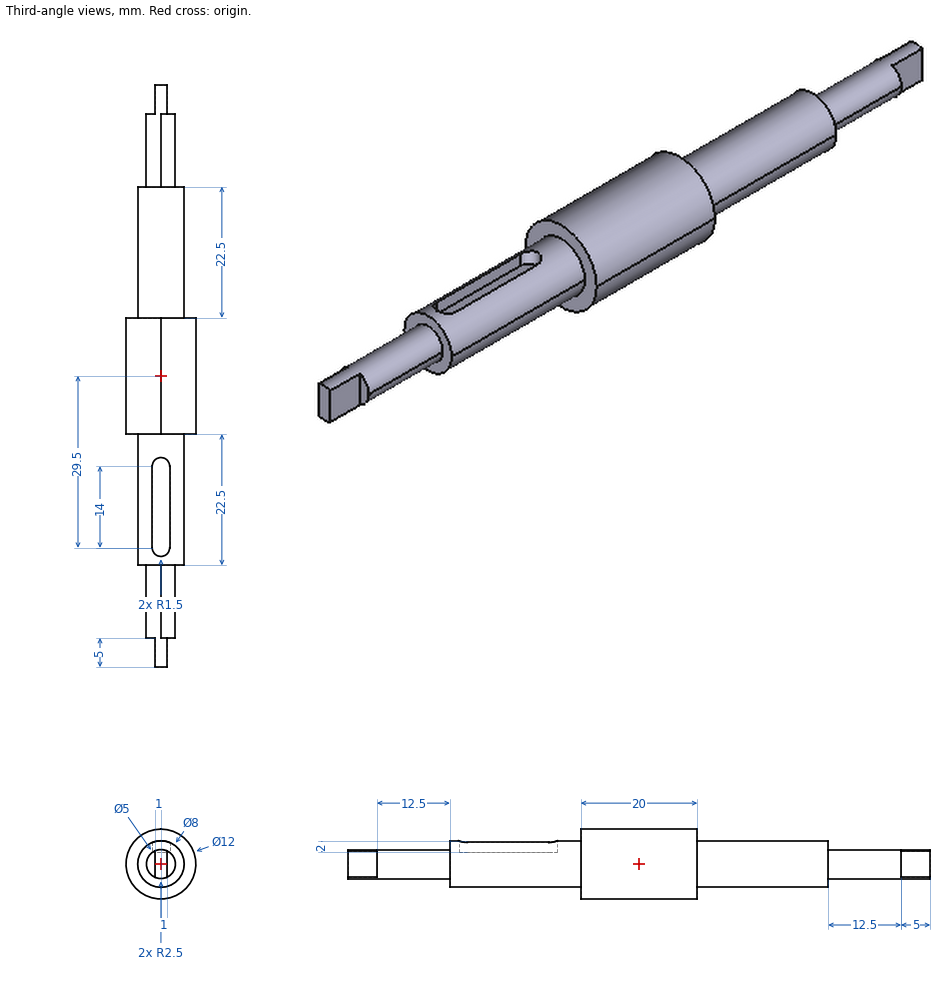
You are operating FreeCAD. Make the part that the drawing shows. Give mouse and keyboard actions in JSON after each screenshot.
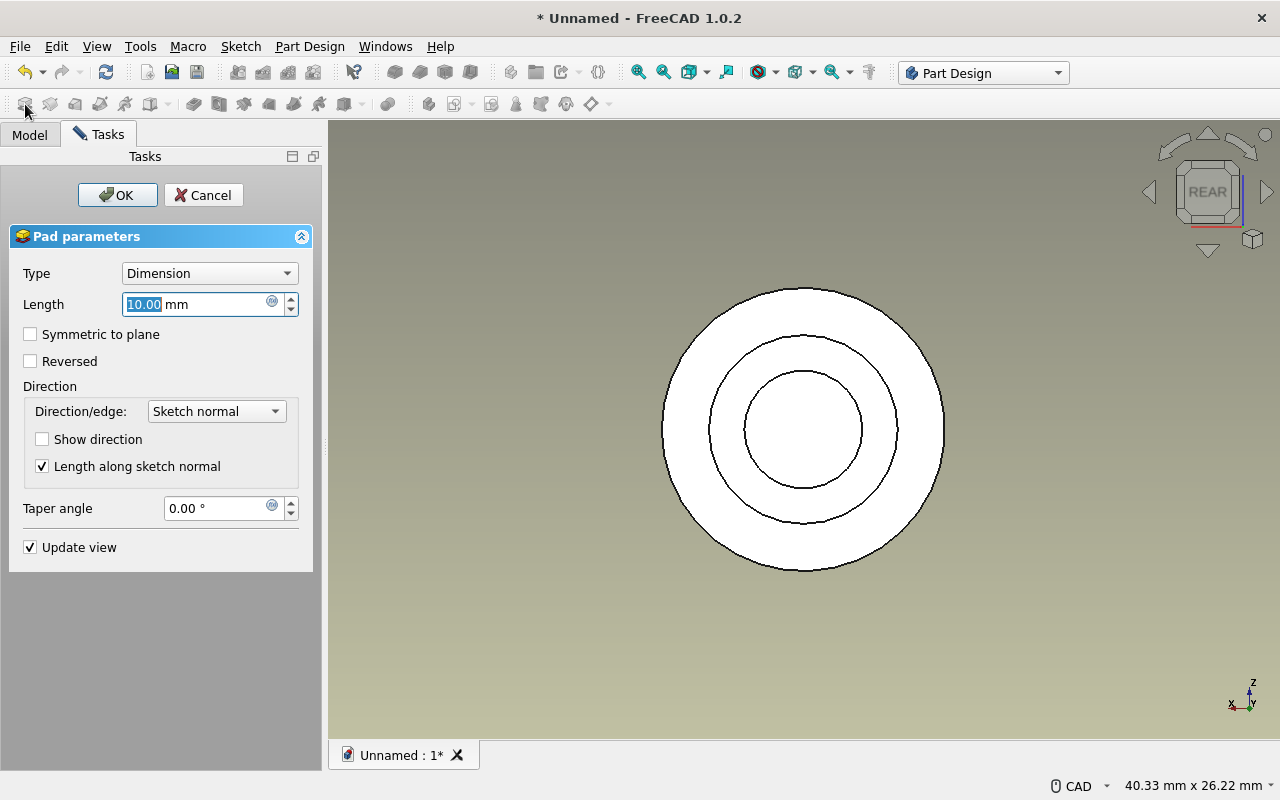
{"action": "type", "text": "22.5"}
{"action": "key", "text": "Tab"}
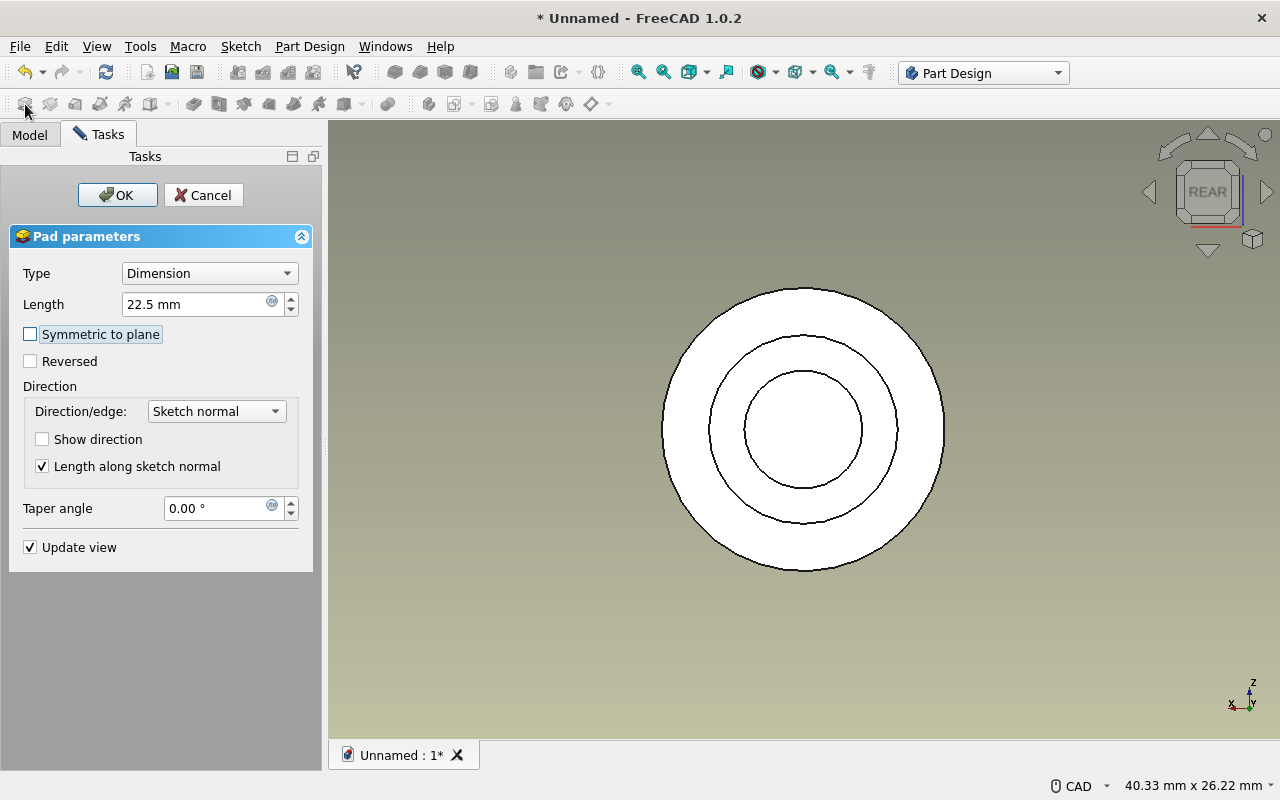
{"action": "left_click", "coordinate": [31, 361]}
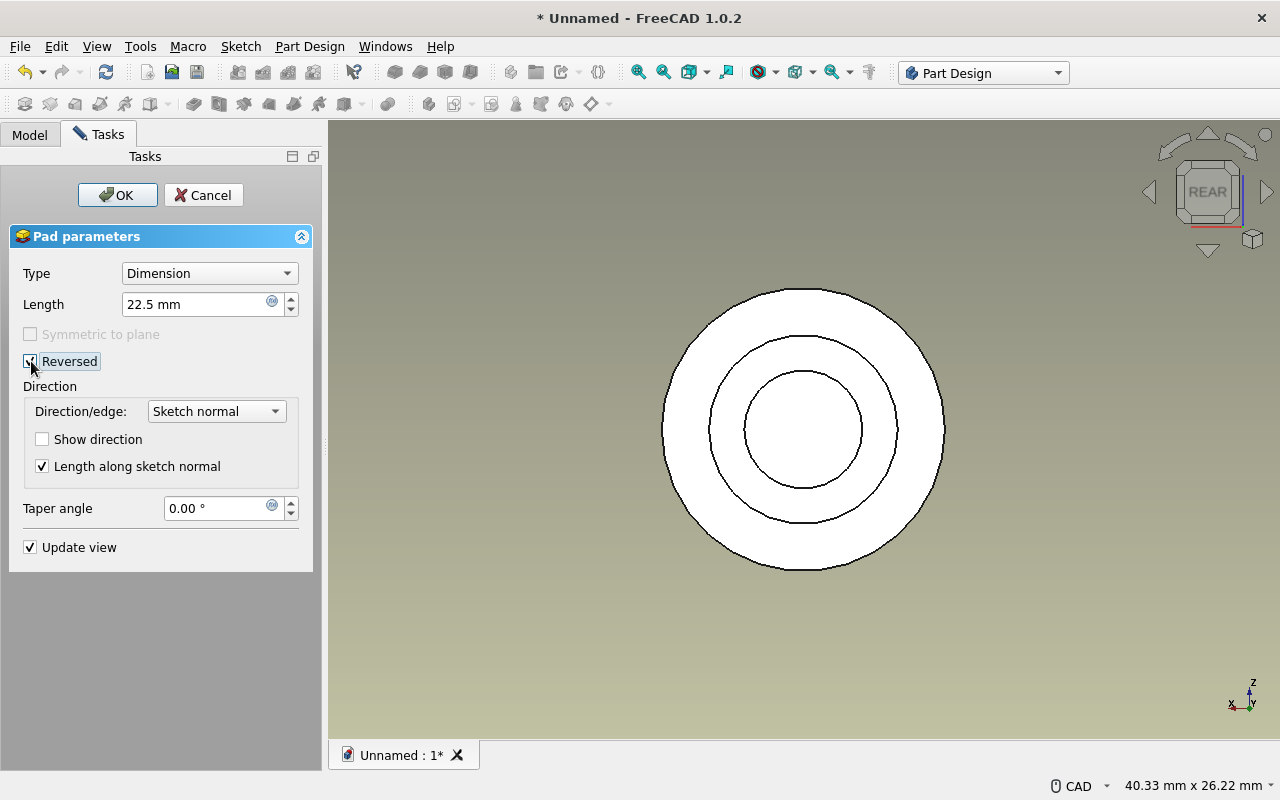
{"action": "left_click", "coordinate": [118, 195]}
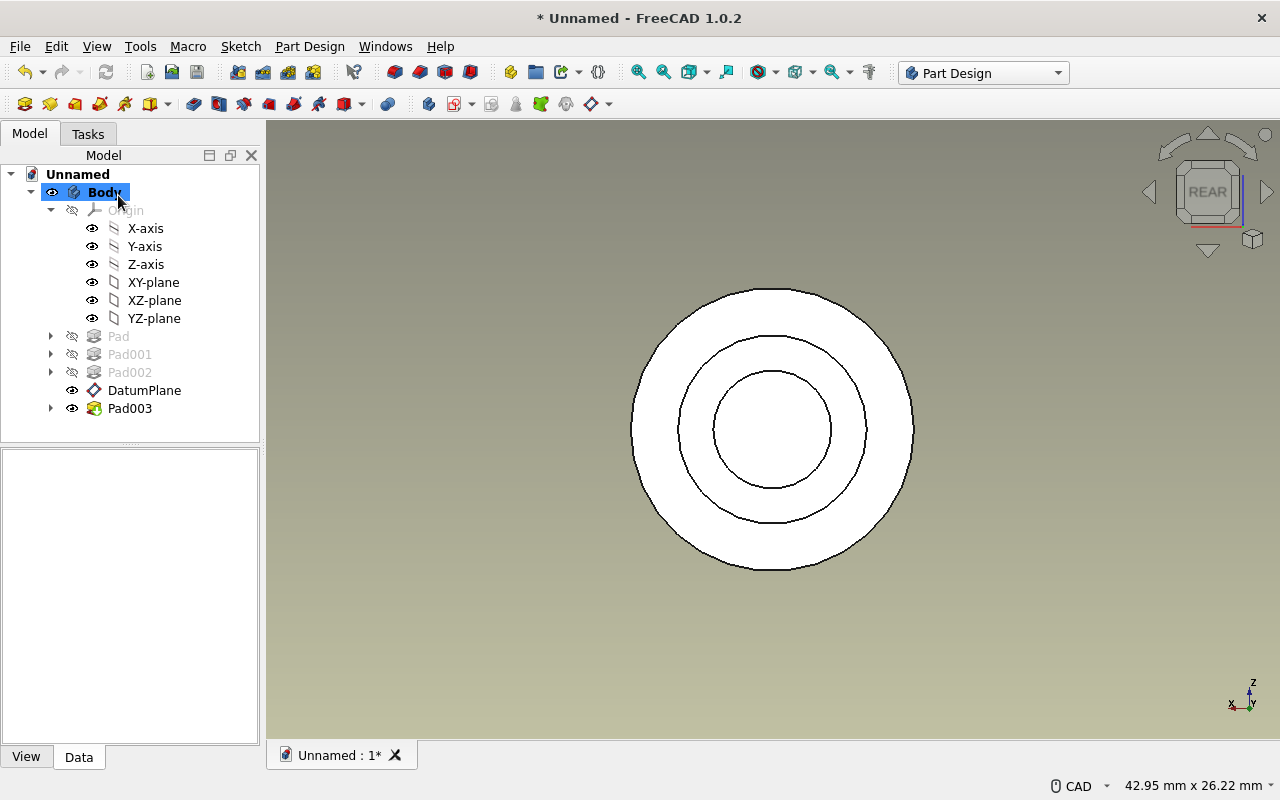
{"action": "left_click", "coordinate": [117, 390]}
{"action": "key", "text": "space"}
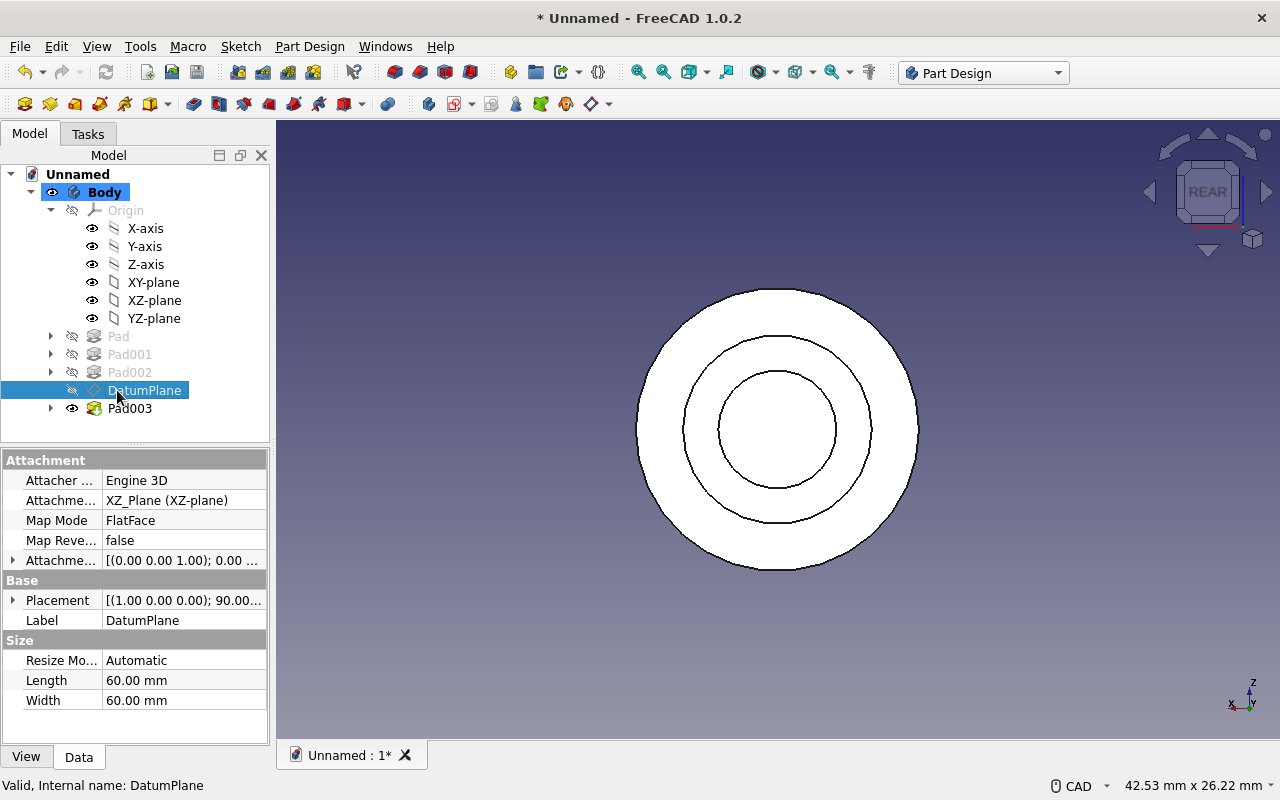
{"action": "left_click", "coordinate": [137, 300]}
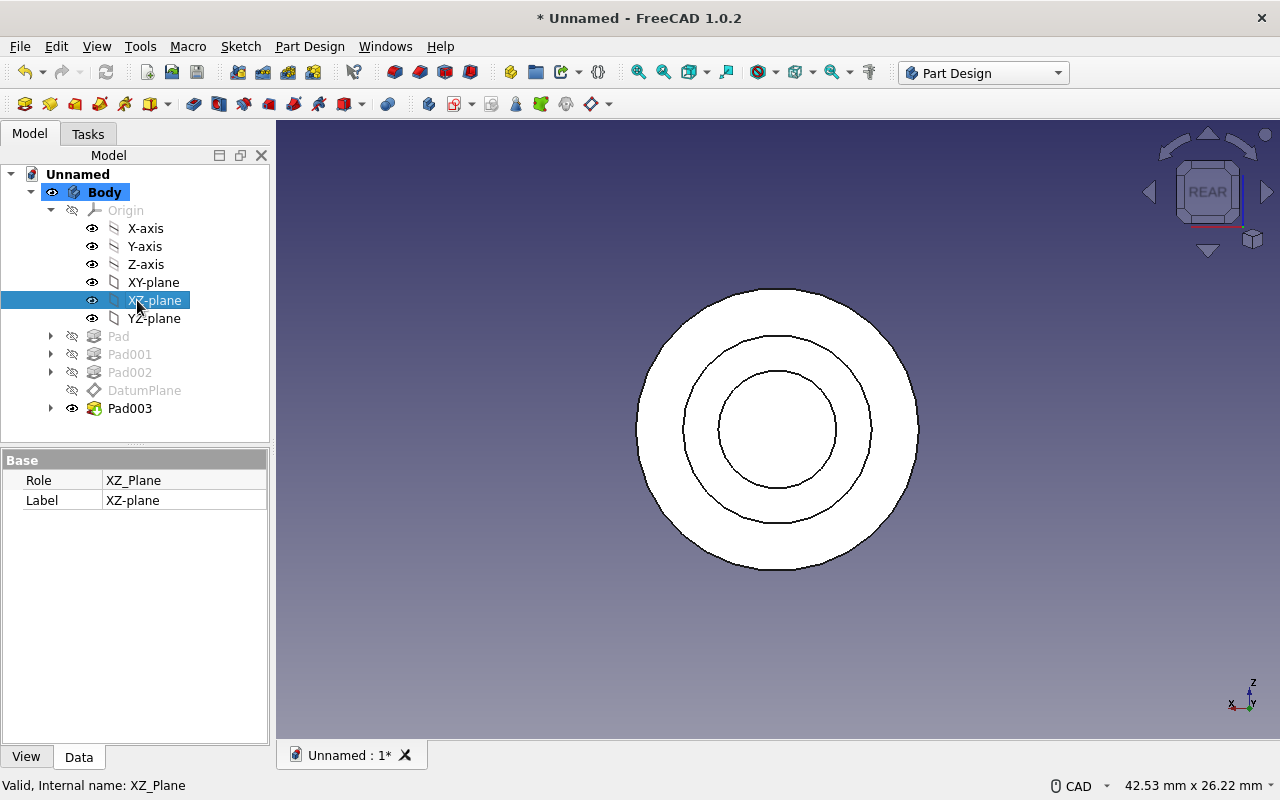
{"action": "left_click", "coordinate": [590, 104]}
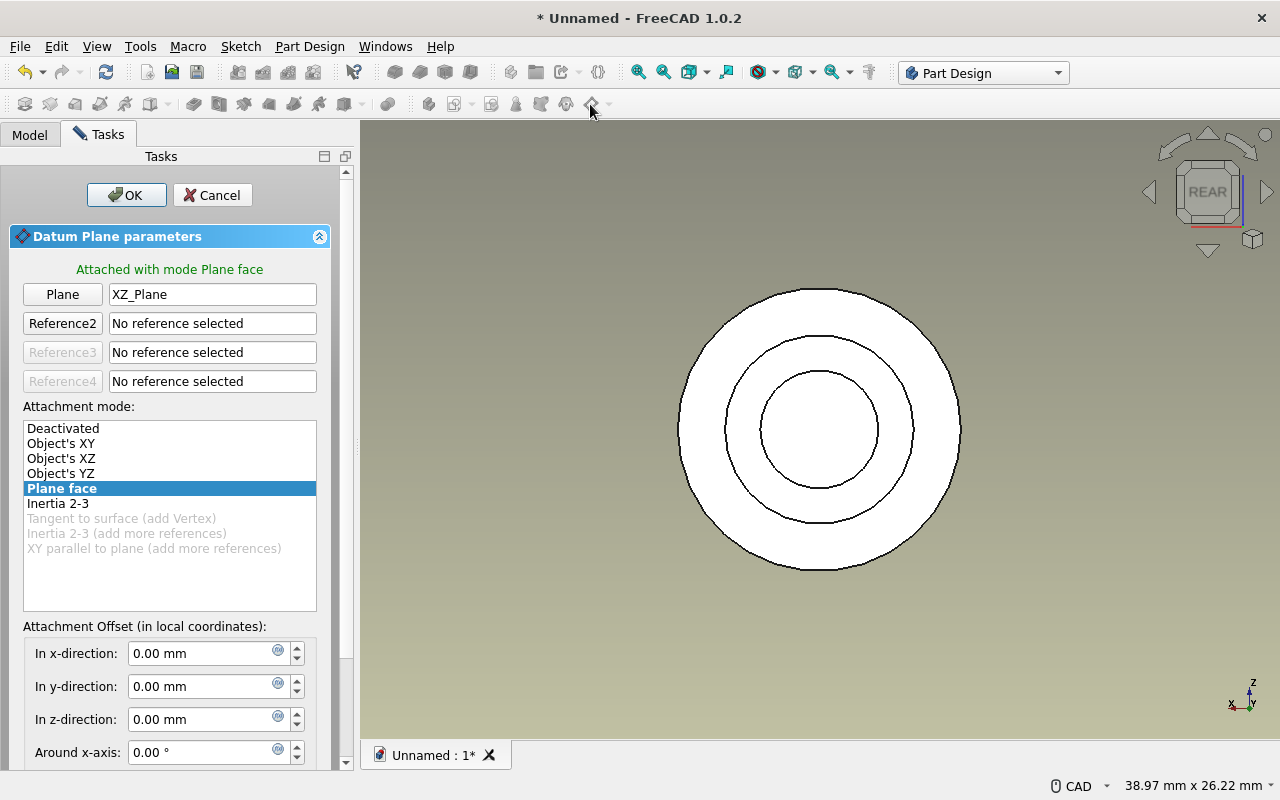
{"action": "triple_click", "coordinate": [210, 720]}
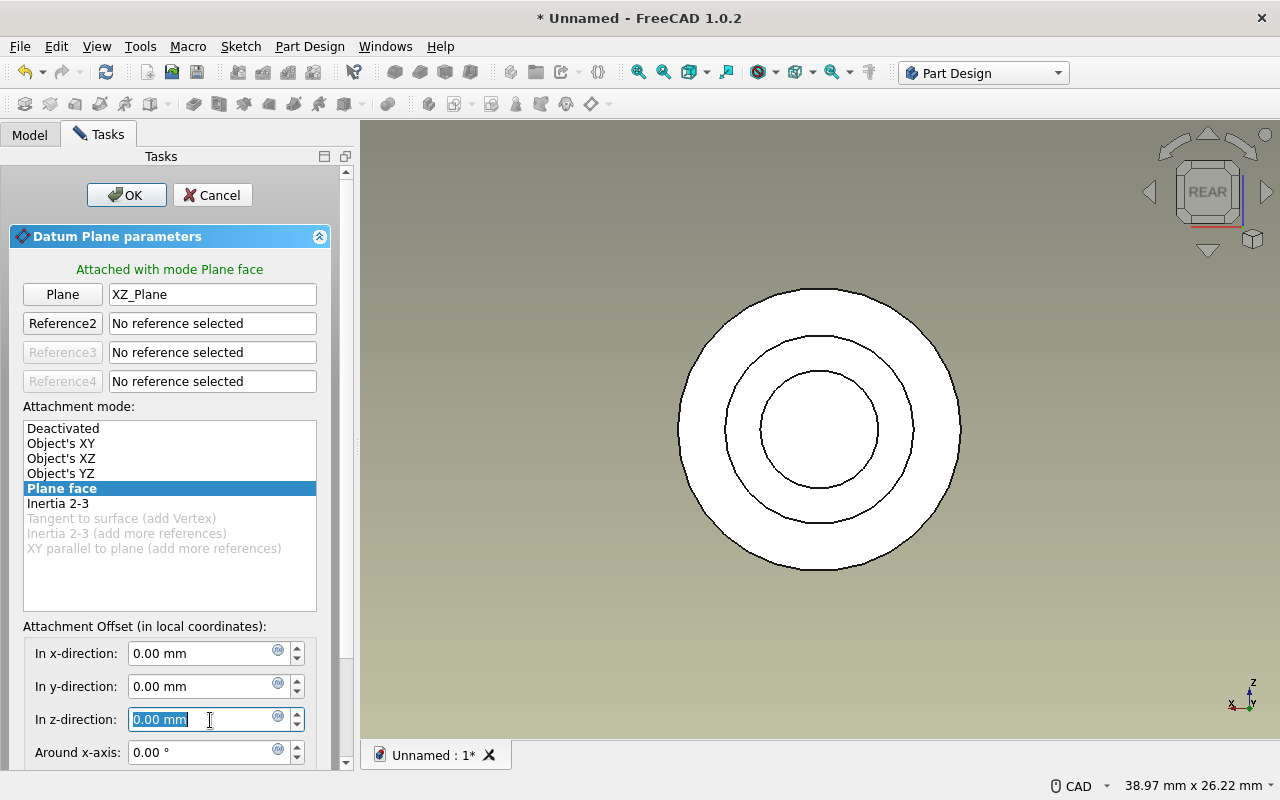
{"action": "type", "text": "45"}
{"action": "key", "text": "Tab"}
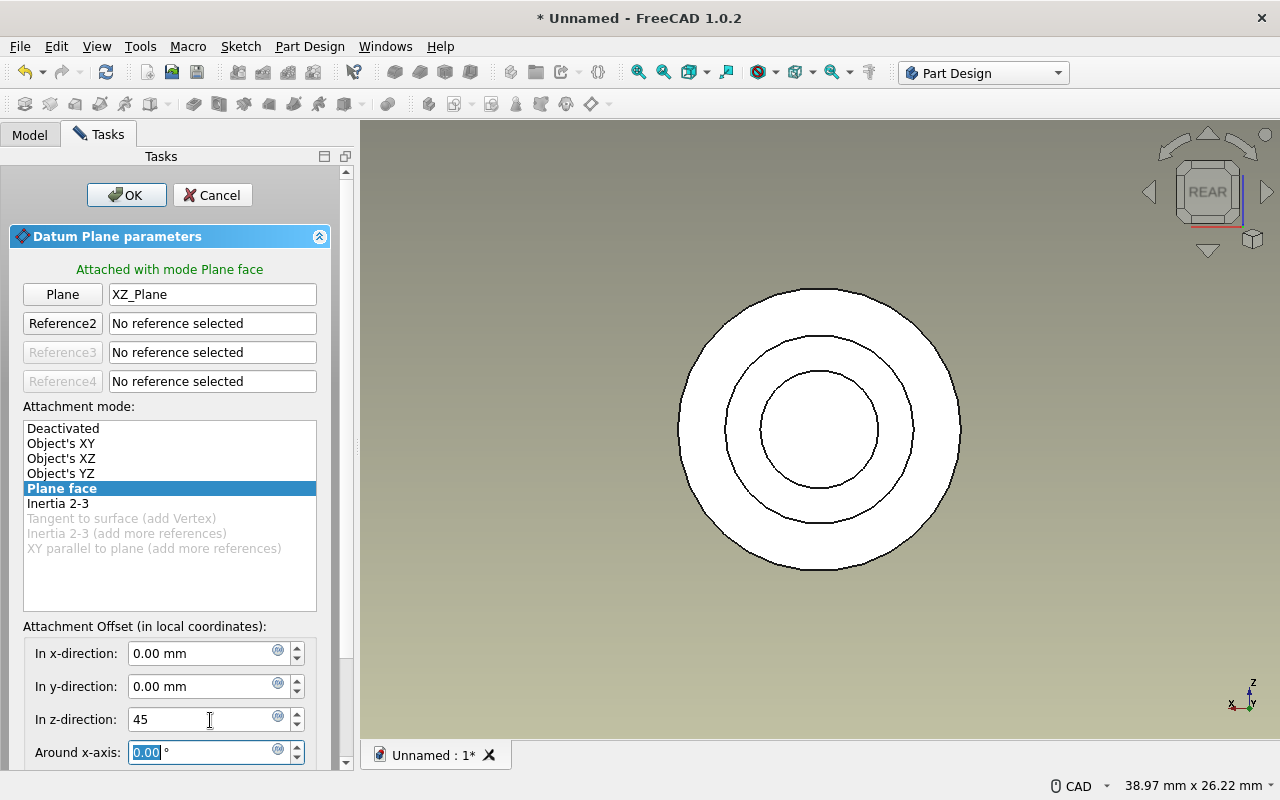
{"action": "left_click", "coordinate": [127, 195]}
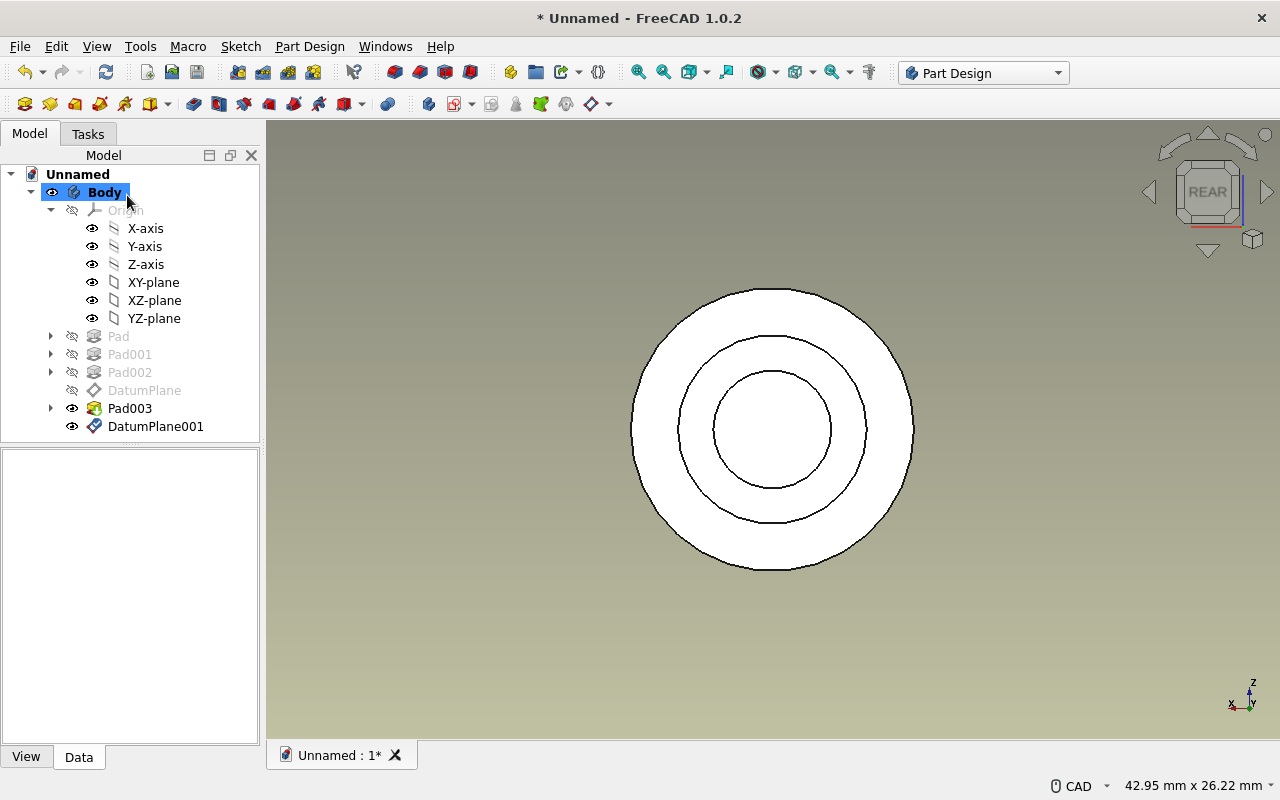
{"action": "left_click", "coordinate": [117, 426]}